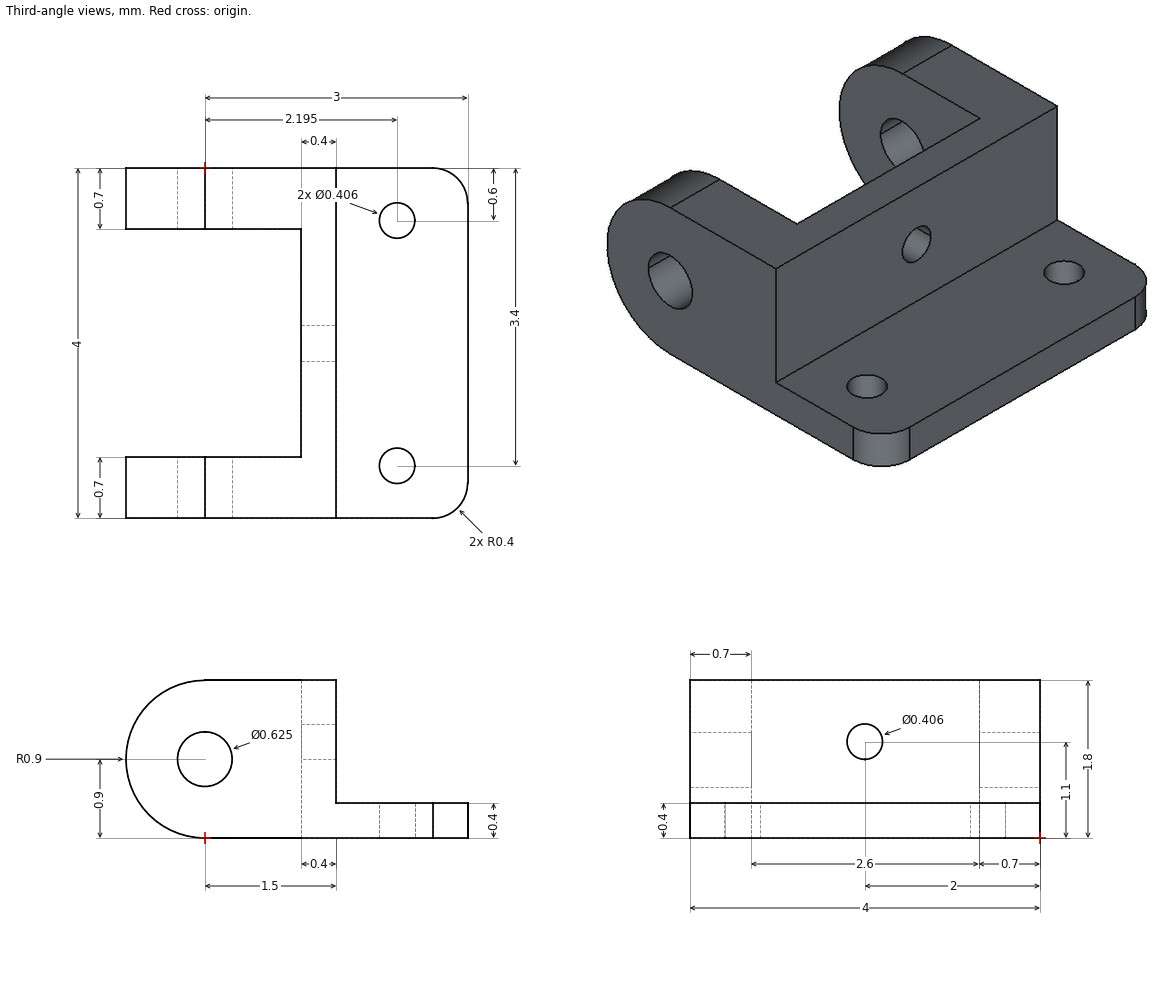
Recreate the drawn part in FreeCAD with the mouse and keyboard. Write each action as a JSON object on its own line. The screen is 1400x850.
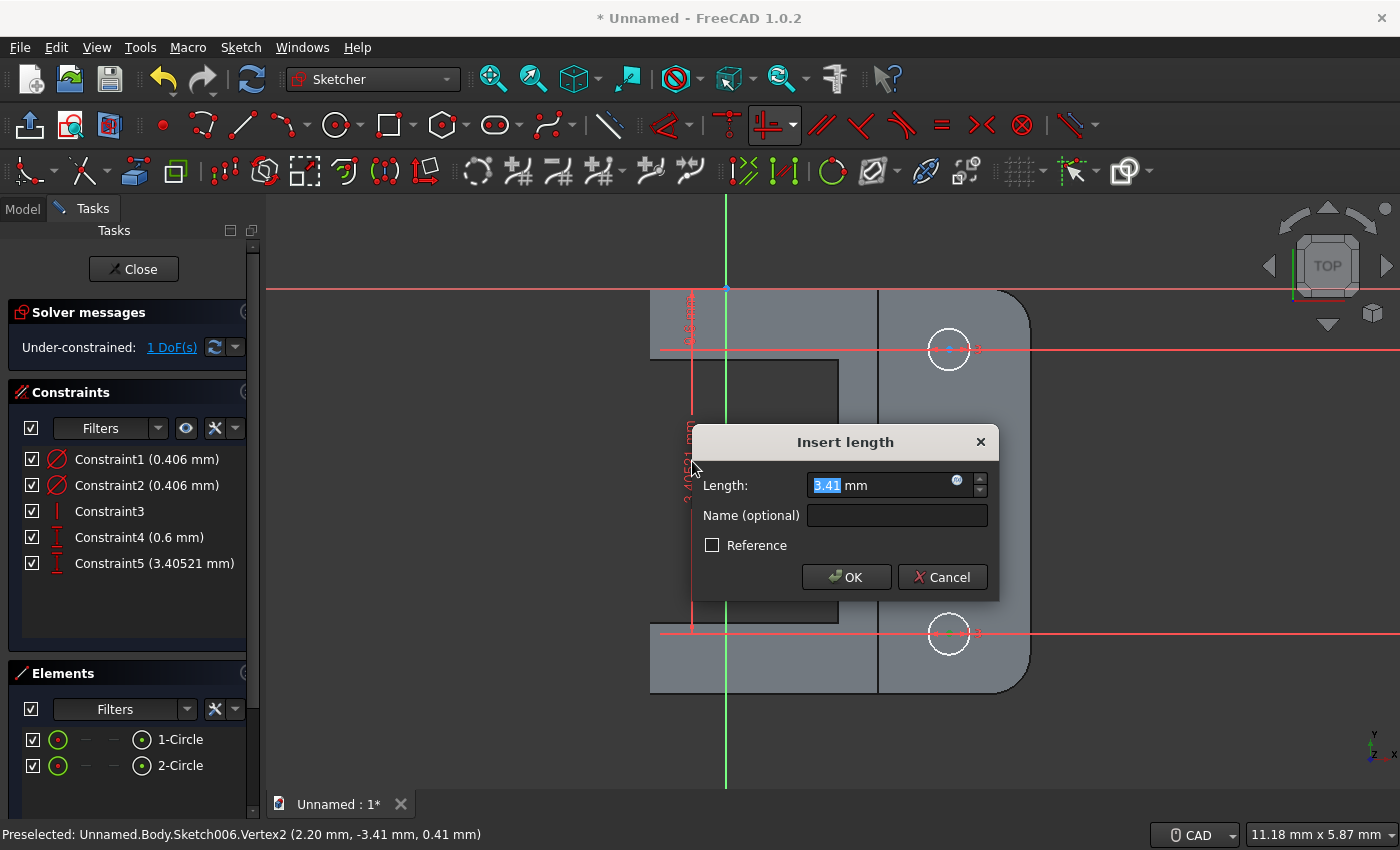
{"action": "type", "text": "3.4"}
{"action": "key", "text": "Return"}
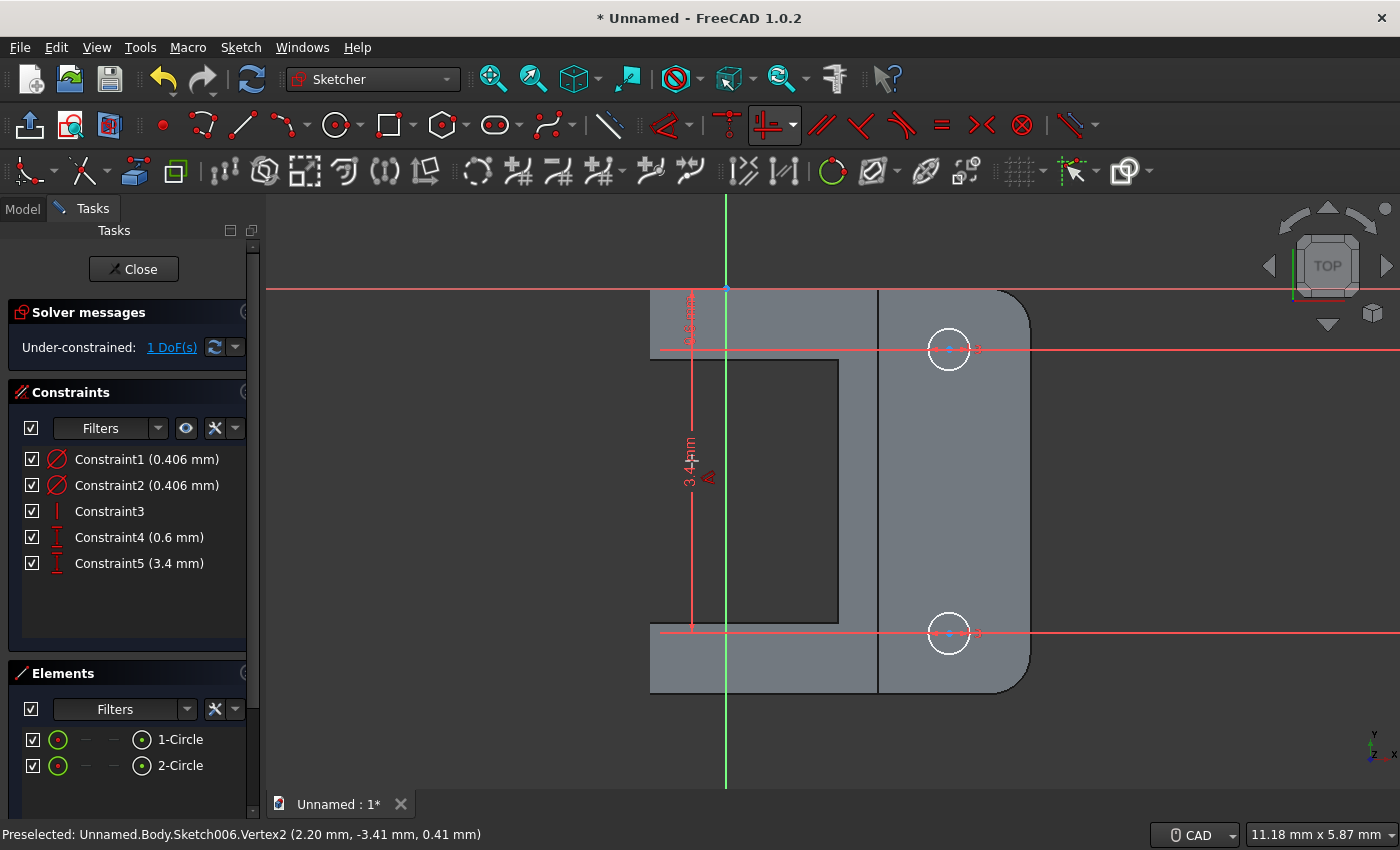
{"action": "left_click", "coordinate": [949, 350]}
{"action": "left_click", "coordinate": [838, 255]}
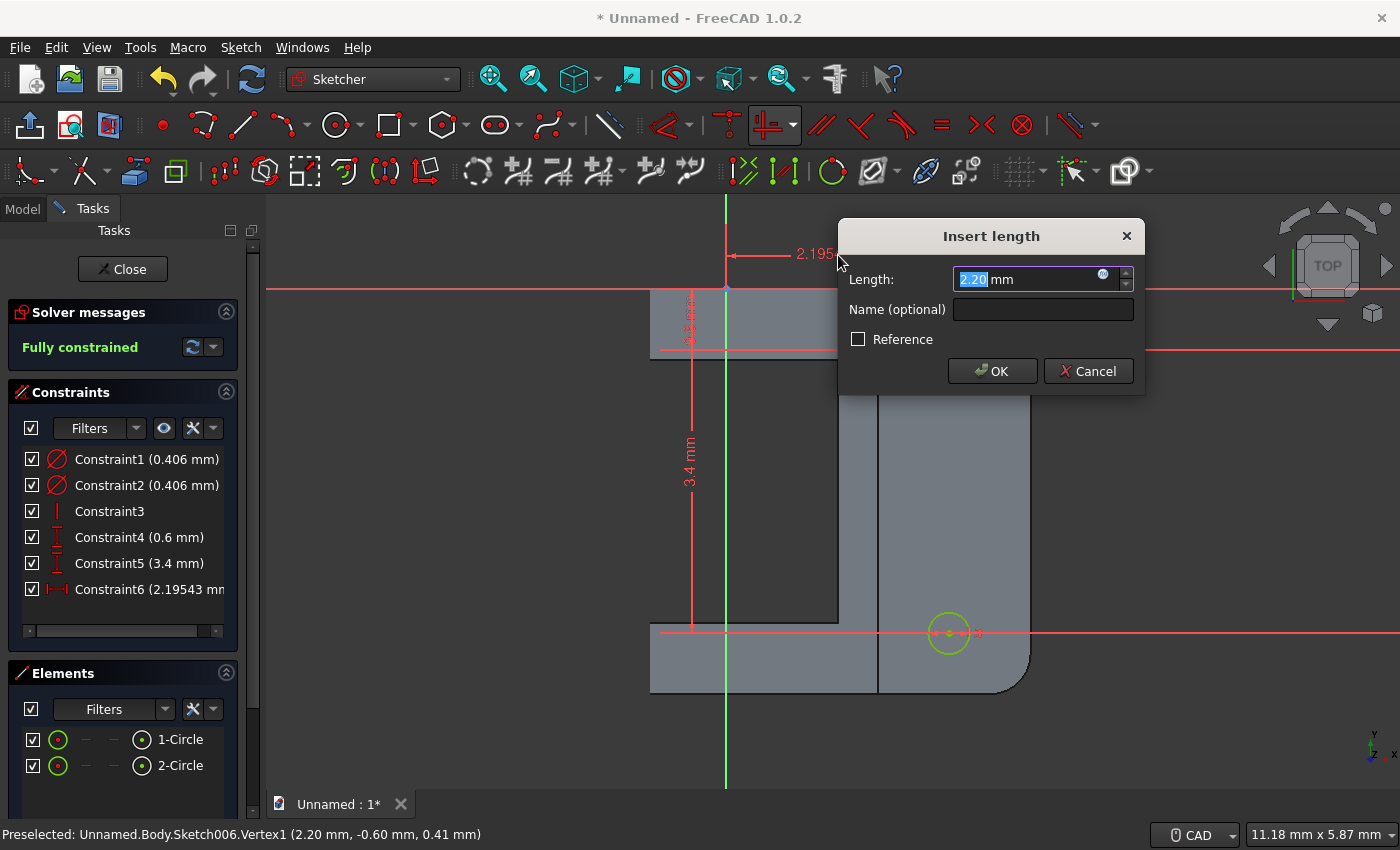
{"action": "type", "text": "2.195"}
{"action": "key", "text": "Return"}
{"action": "key", "text": "Escape"}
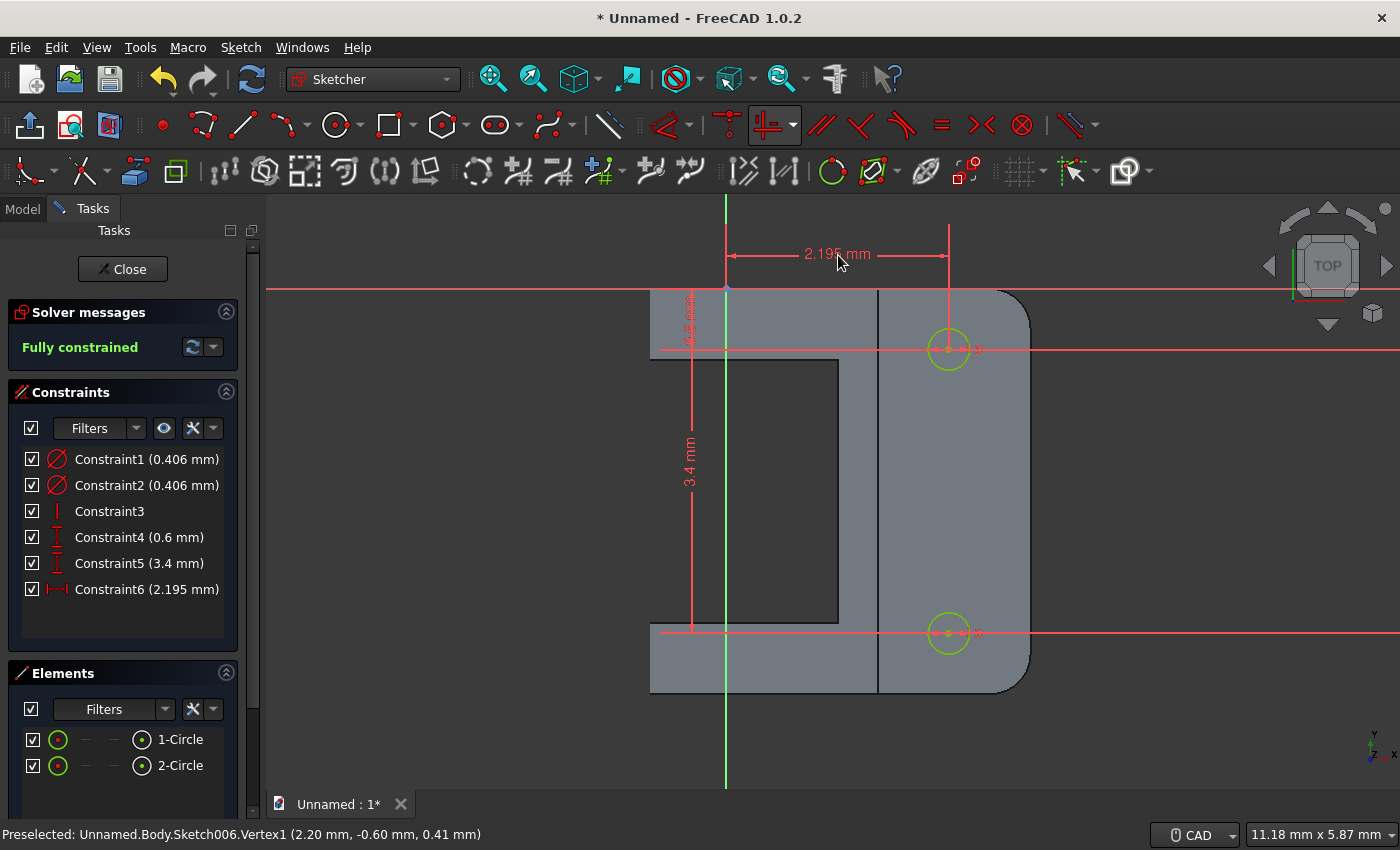
{"action": "left_click", "coordinate": [123, 269]}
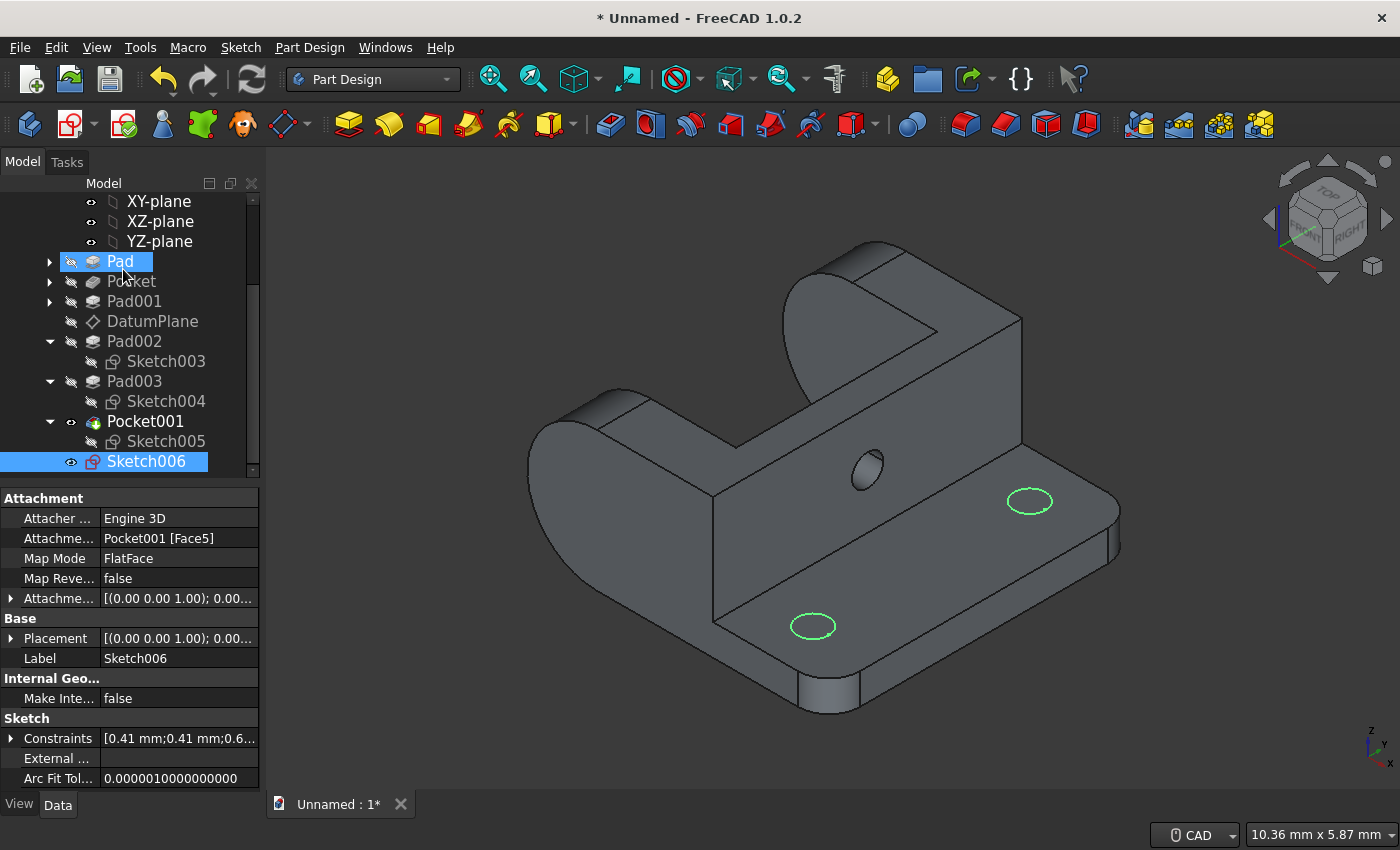
{"action": "left_click", "coordinate": [612, 124]}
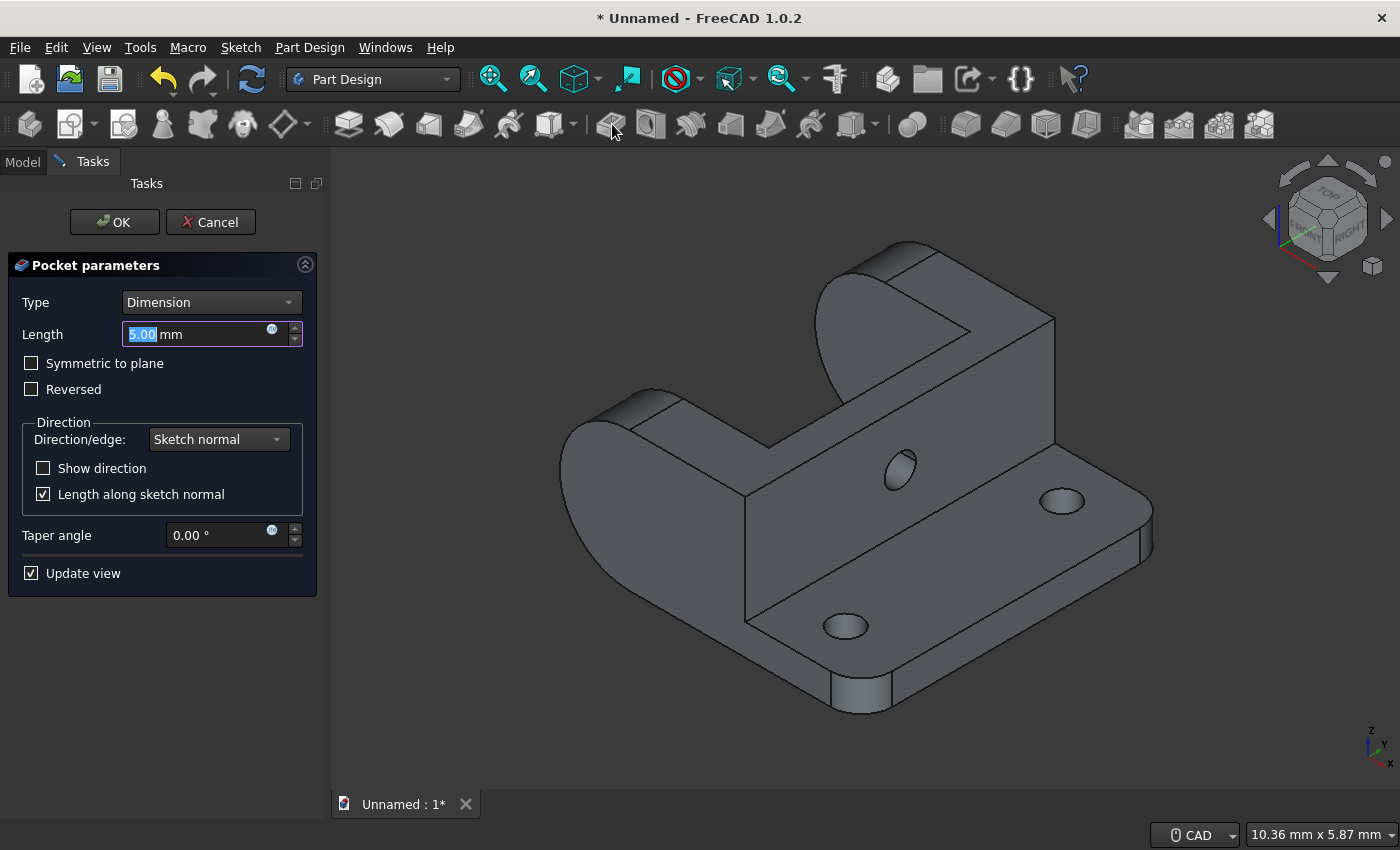
{"action": "type", "text": "0.4"}
{"action": "key", "text": "Tab"}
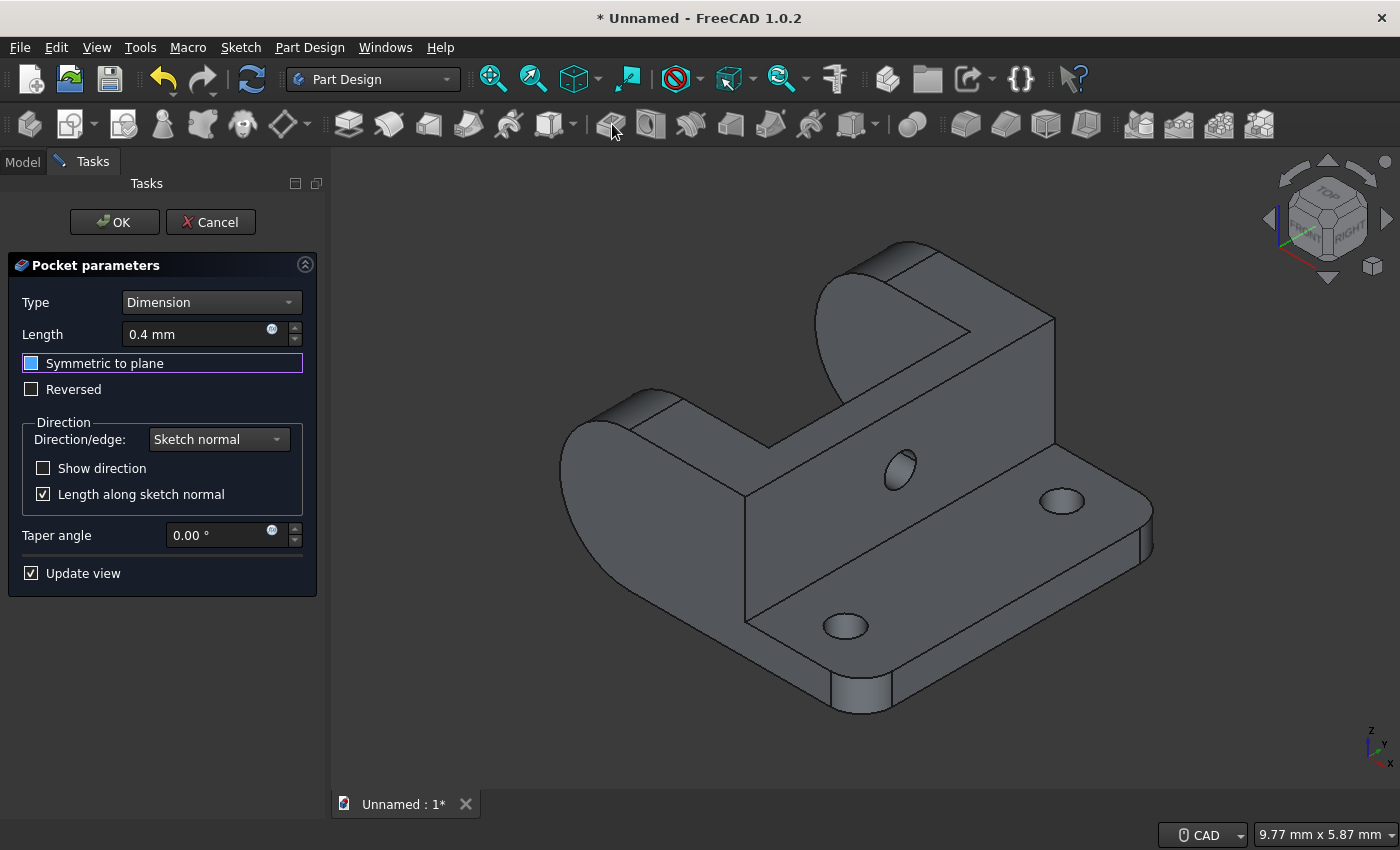
{"action": "left_click", "coordinate": [115, 222]}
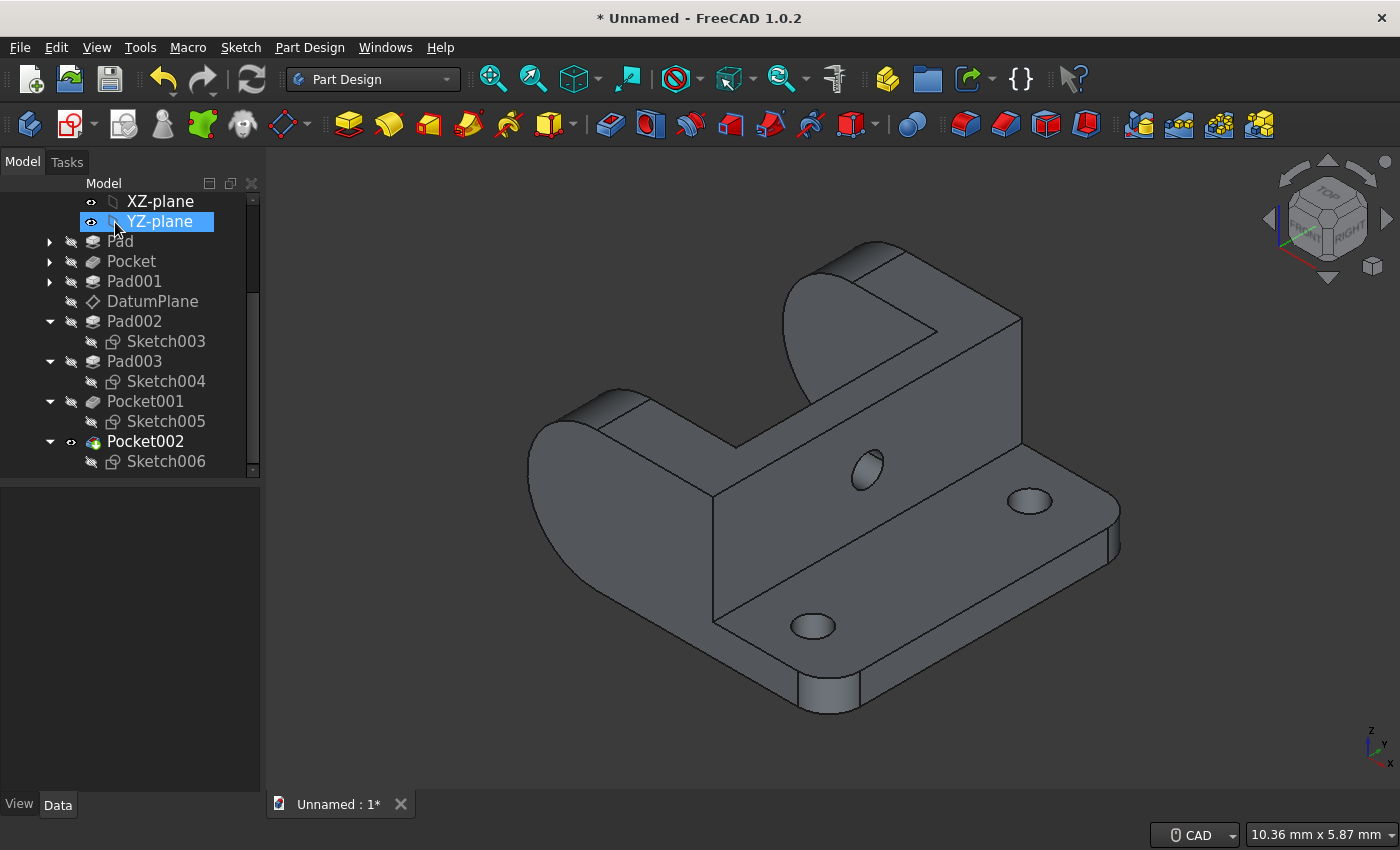
{"action": "key", "text": "4"}